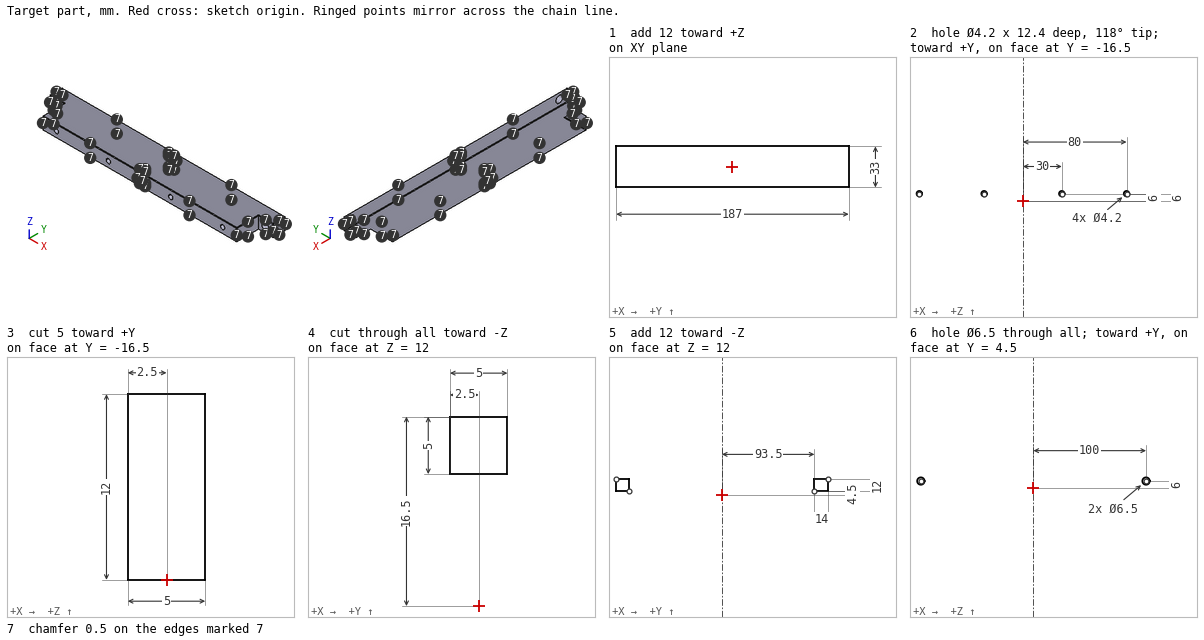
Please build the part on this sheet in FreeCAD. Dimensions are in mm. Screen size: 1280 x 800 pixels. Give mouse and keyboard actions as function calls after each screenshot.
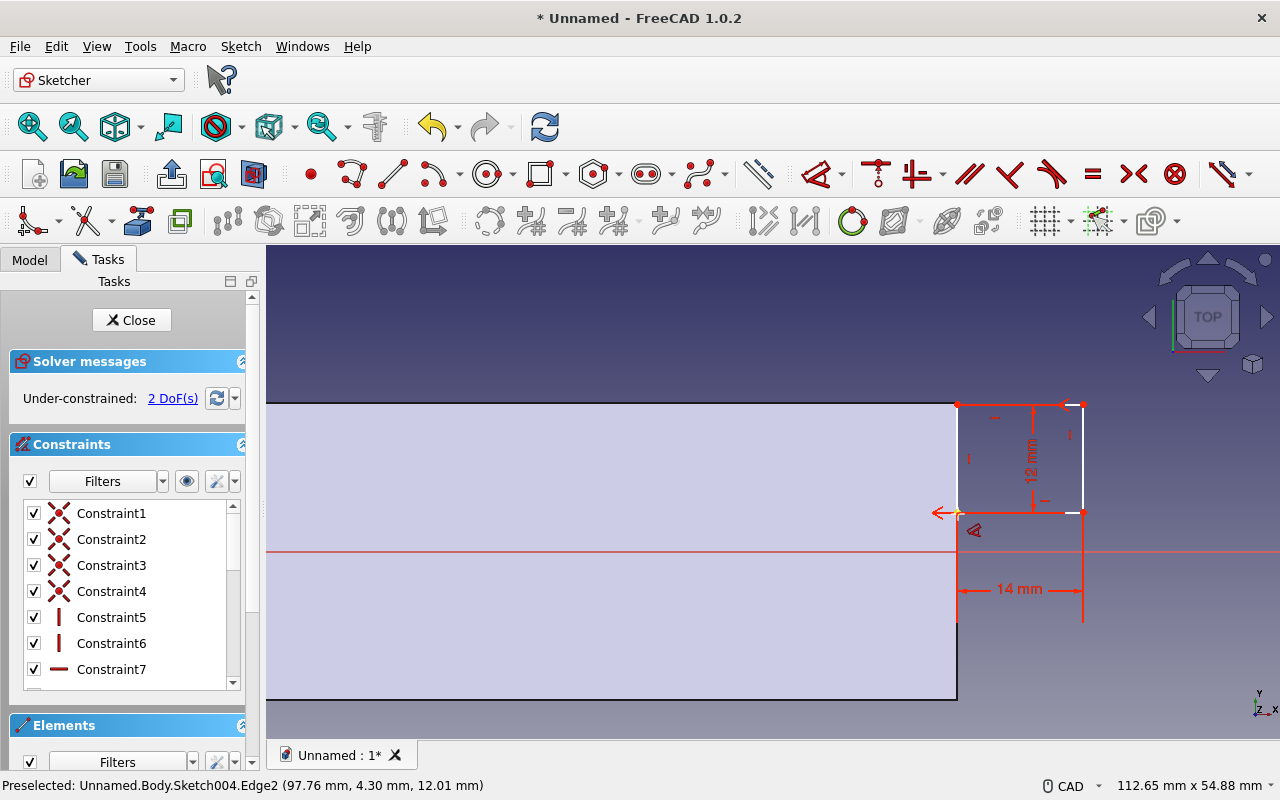
click(957, 513)
click(991, 532)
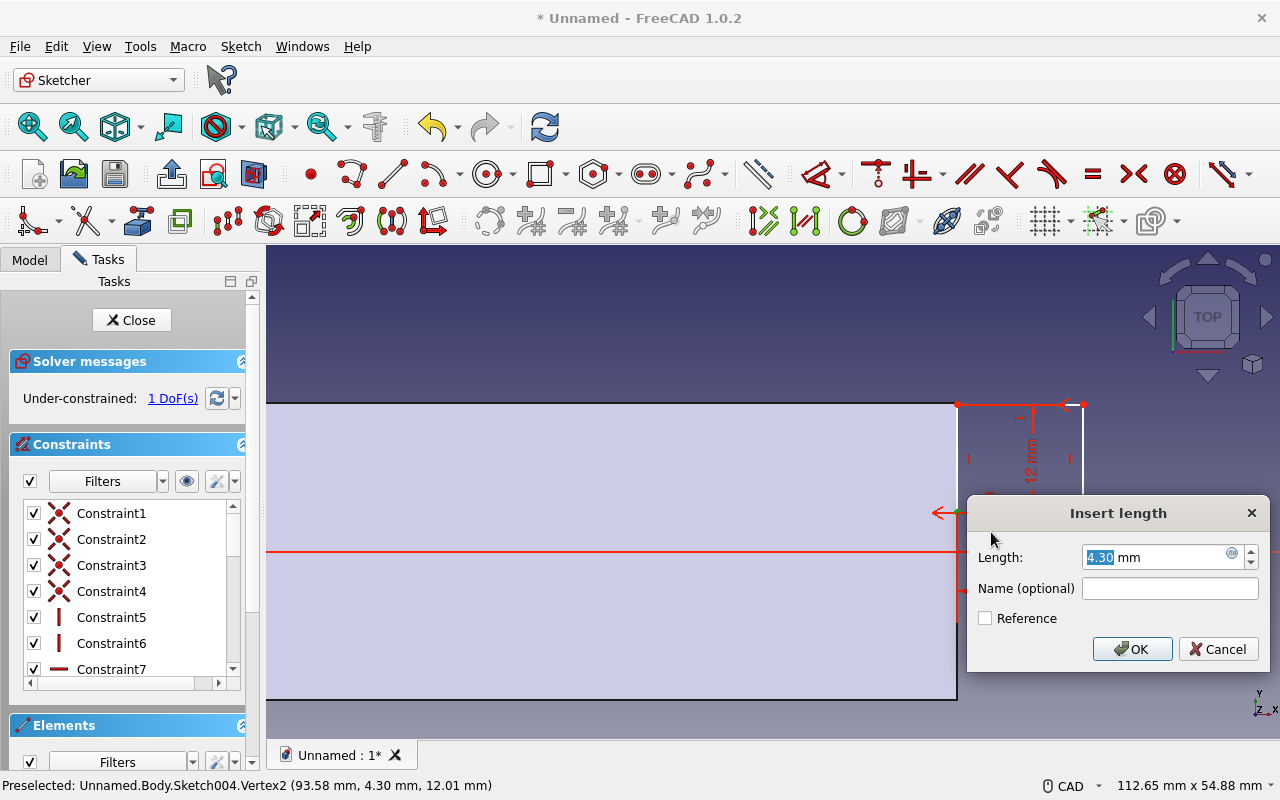
text(4.5)
key(Return)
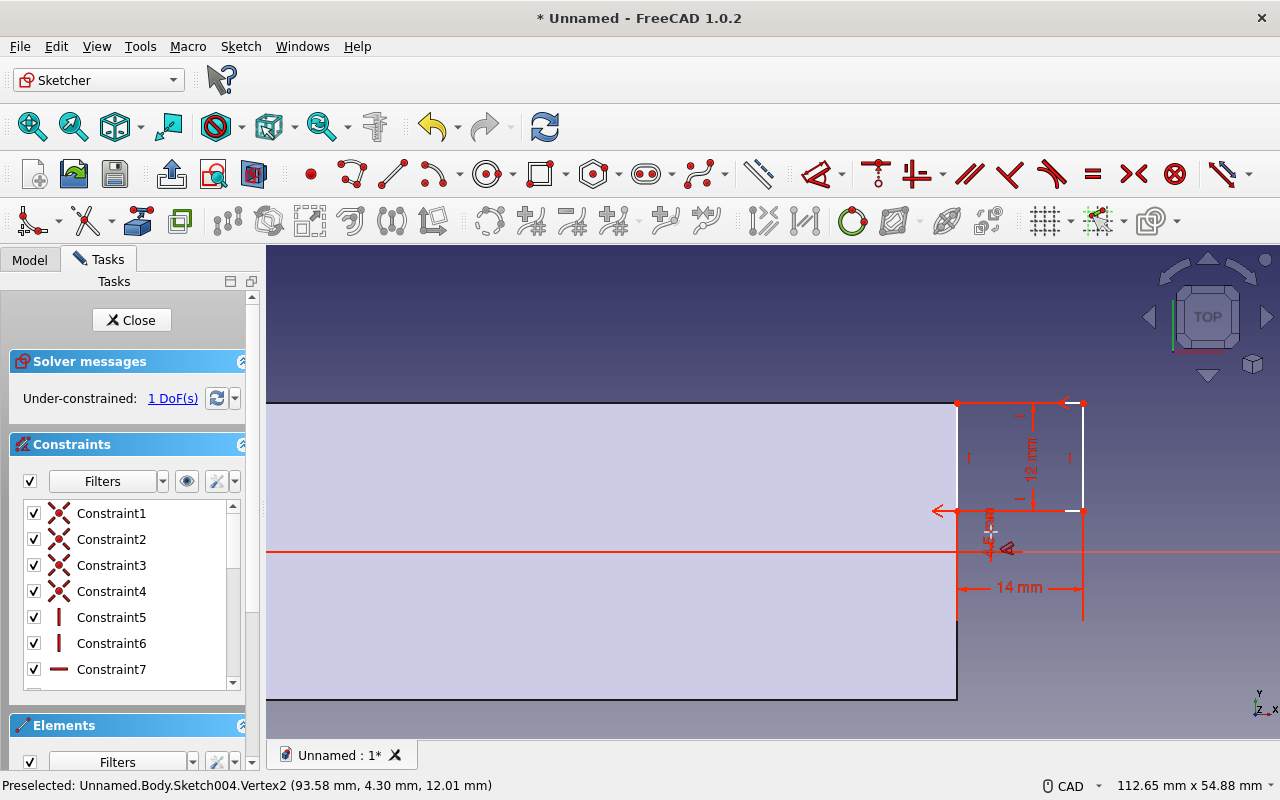
click(957, 403)
click(626, 586)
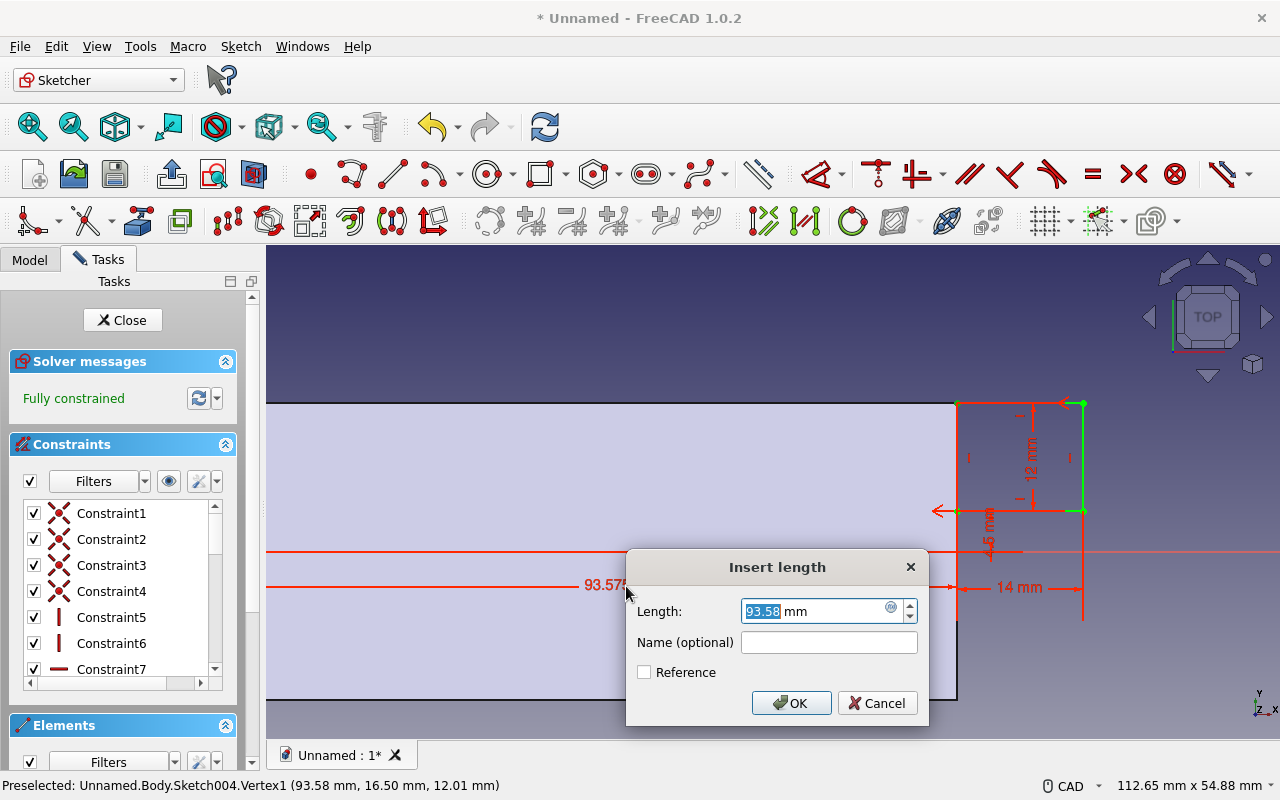
text(93.5)
key(Return)
key(Escape)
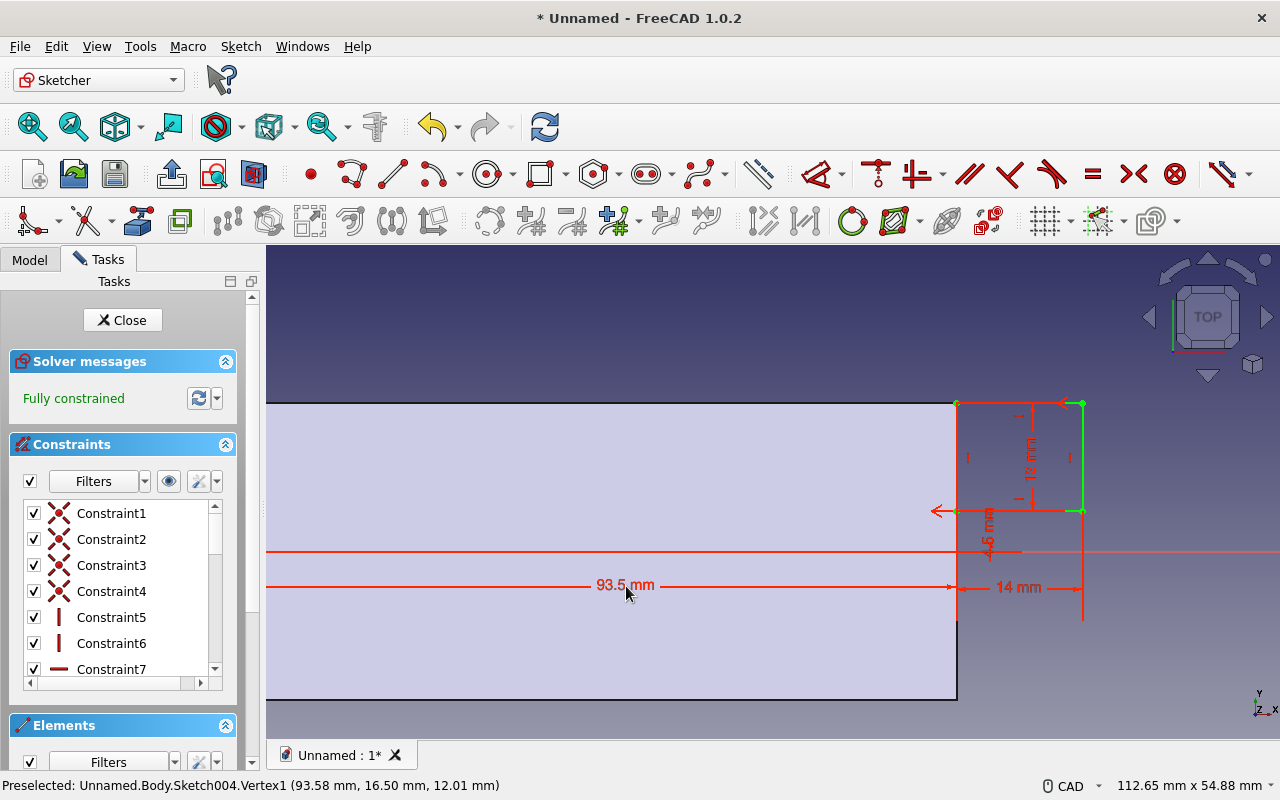
click(123, 320)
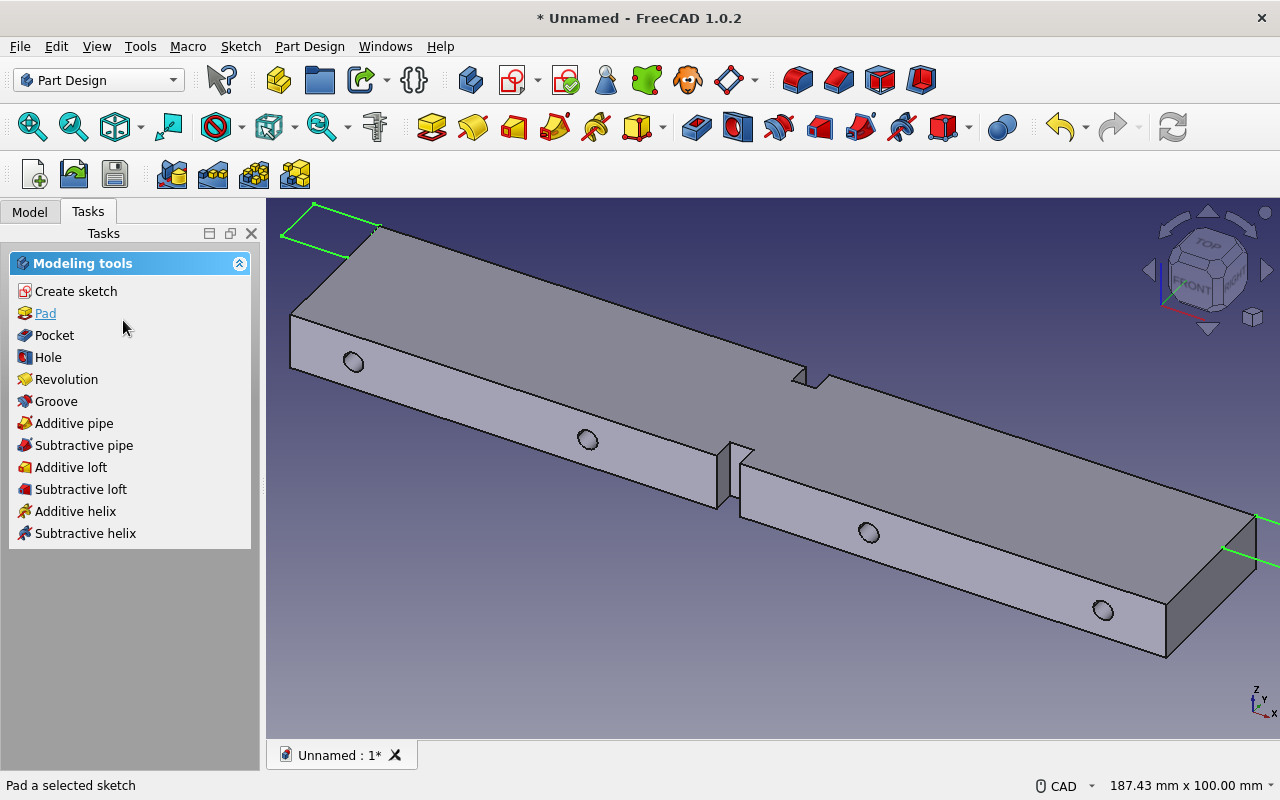
click(432, 128)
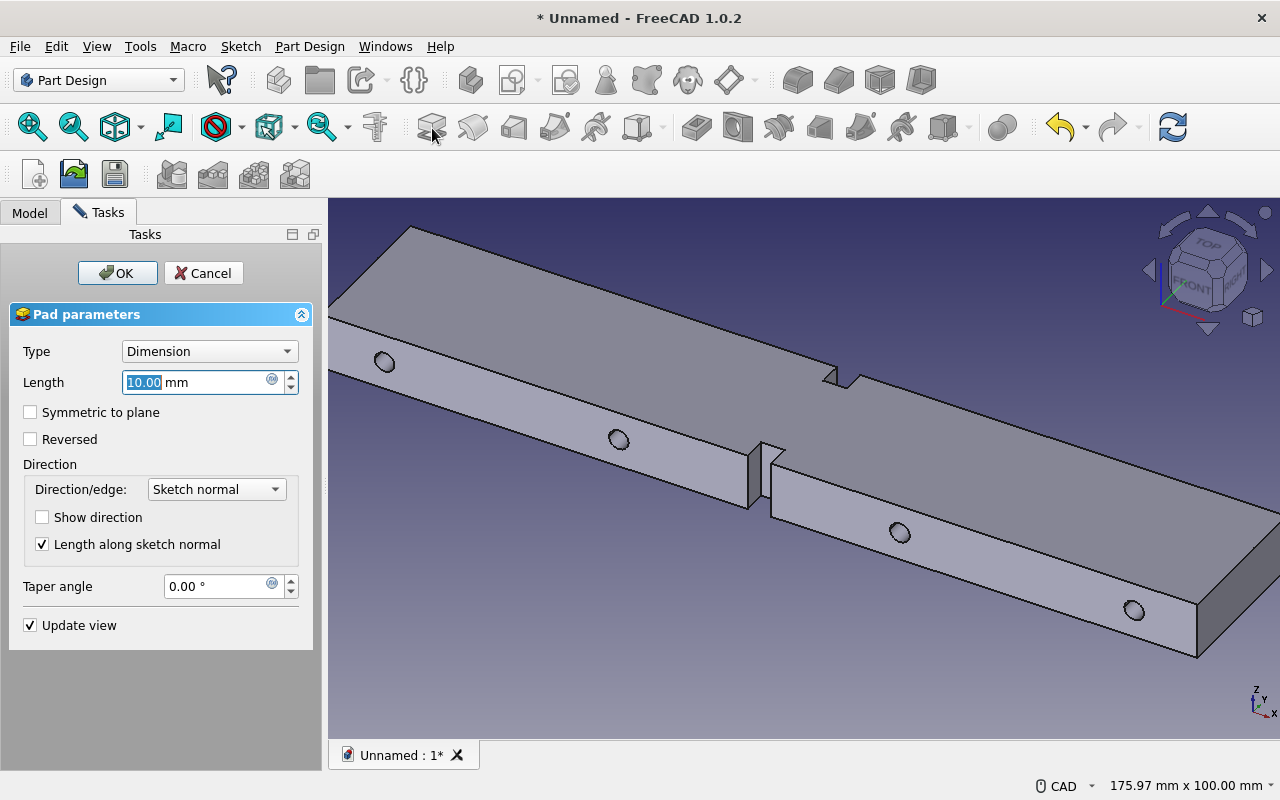
text(12)
key(Tab)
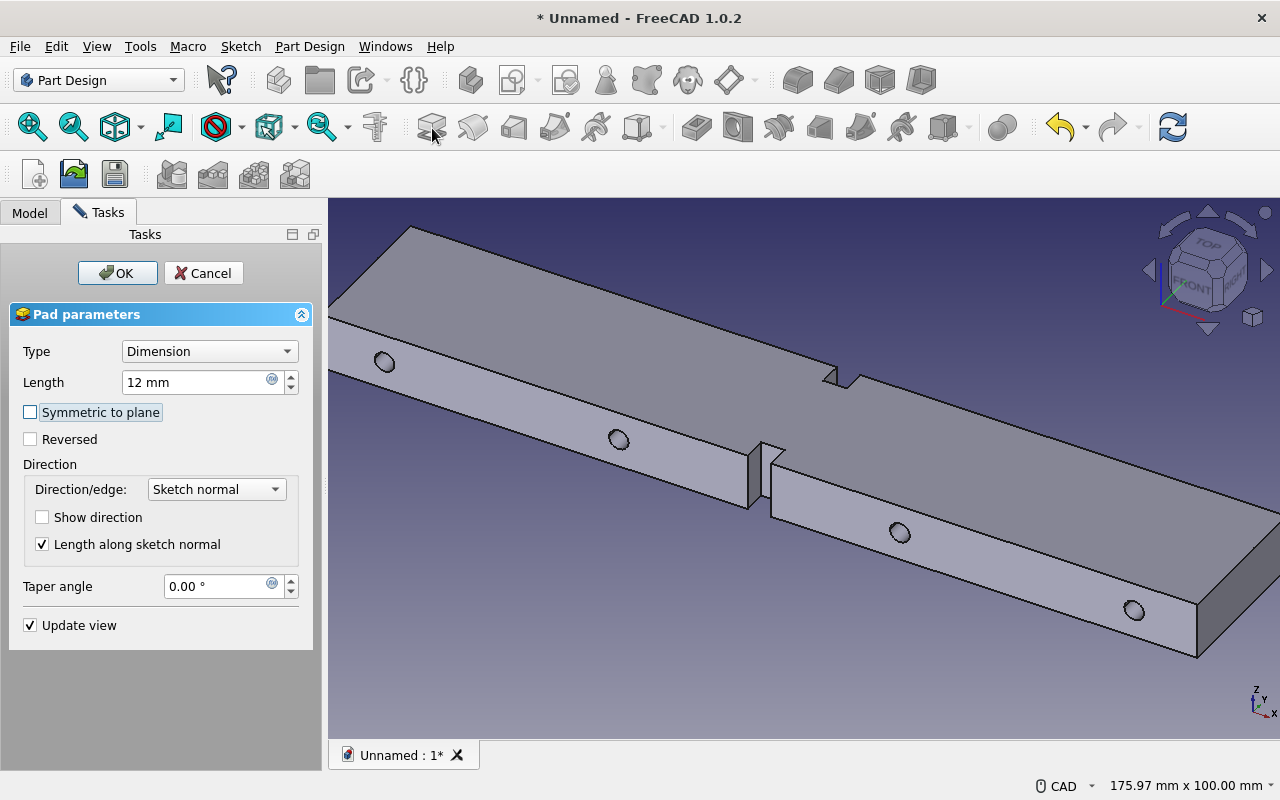
click(31, 439)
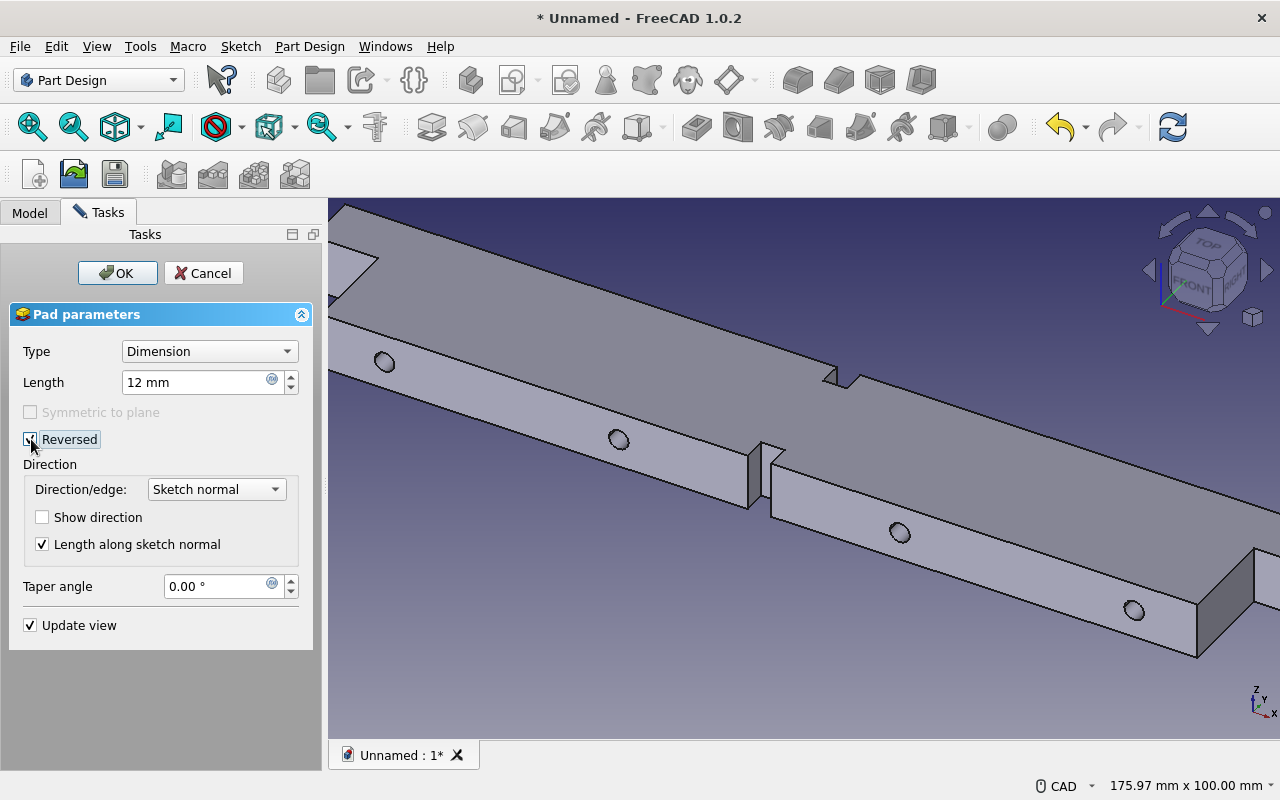
click(118, 273)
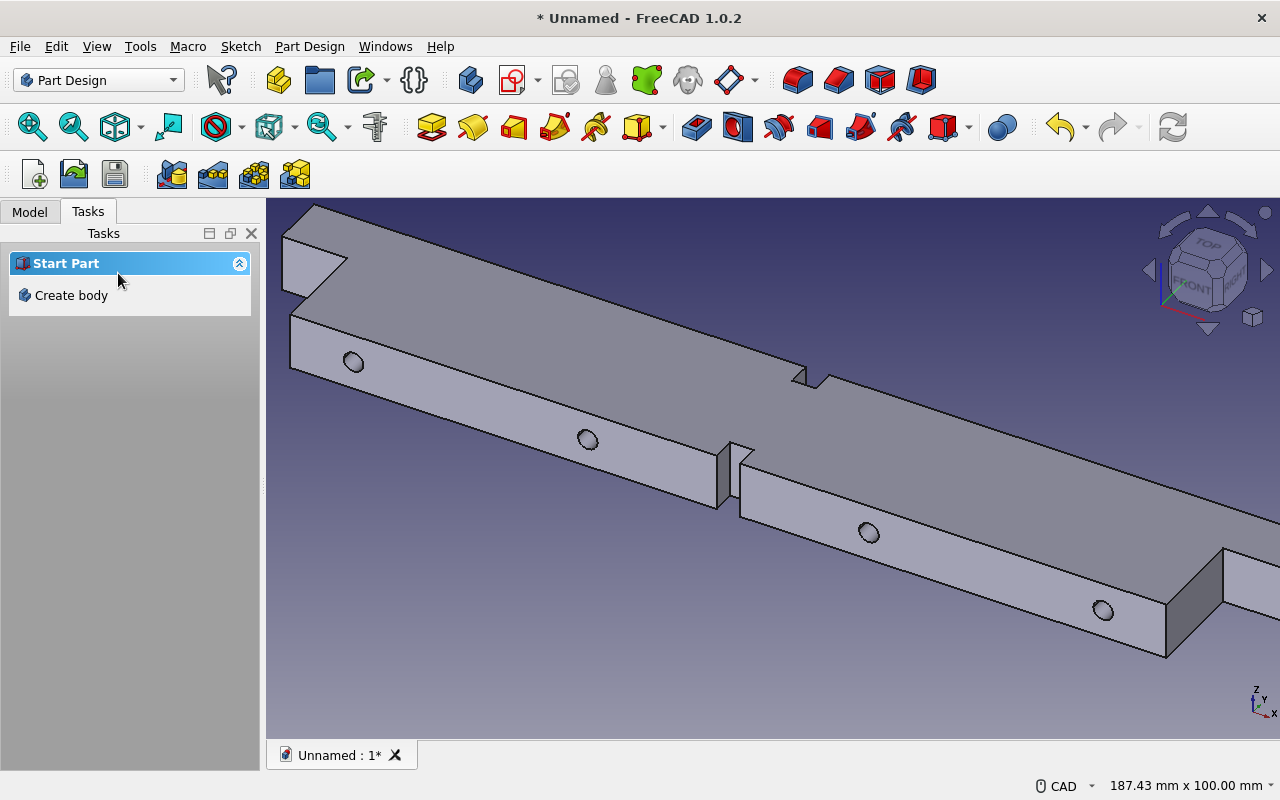
key(v)
key(f)